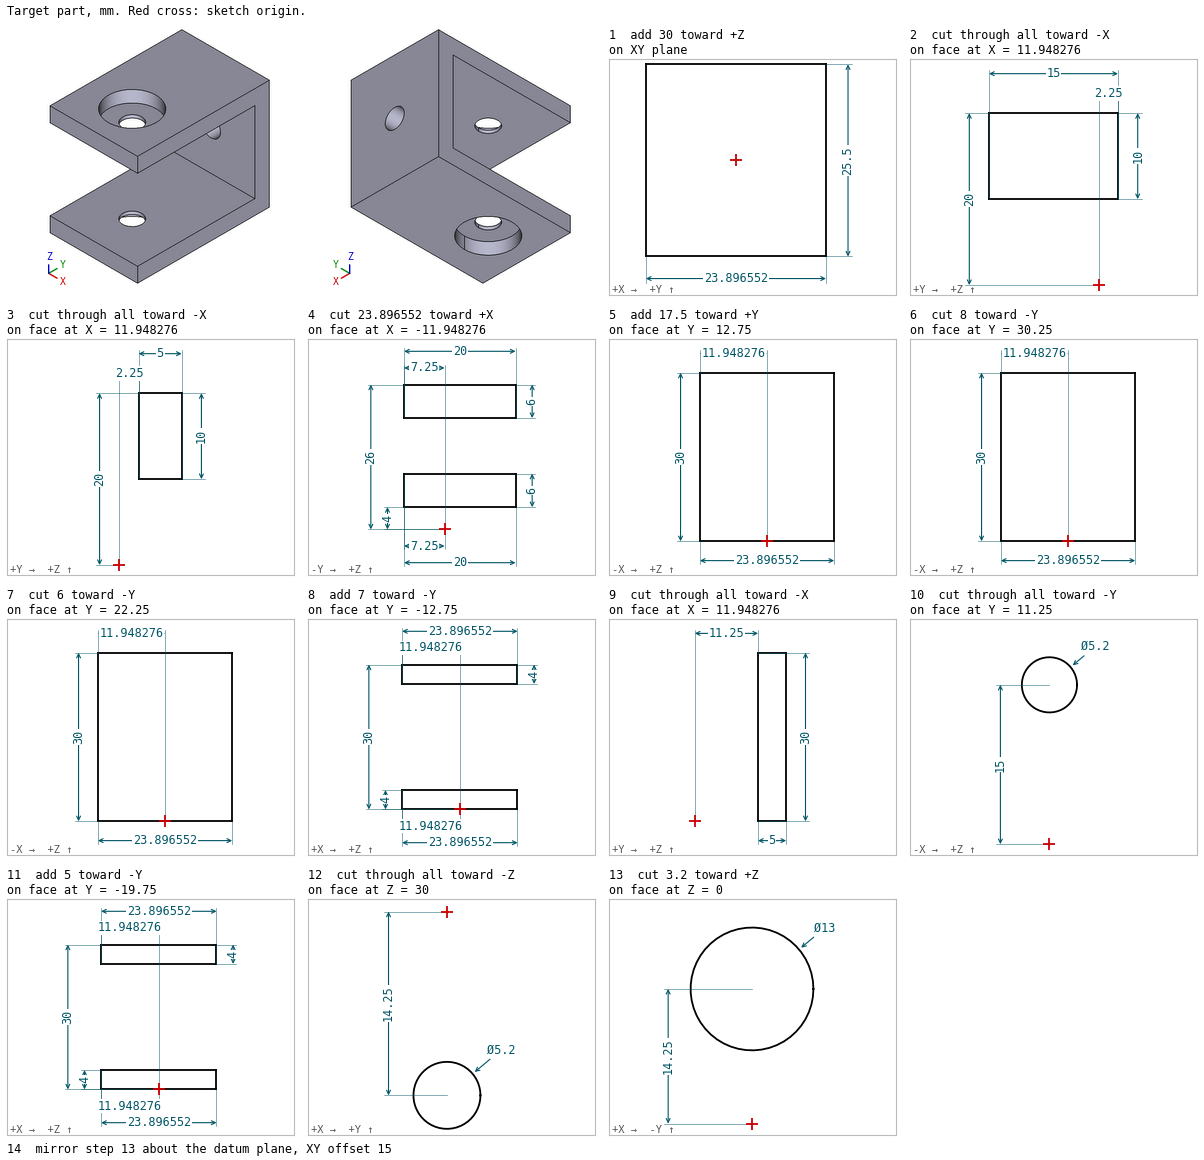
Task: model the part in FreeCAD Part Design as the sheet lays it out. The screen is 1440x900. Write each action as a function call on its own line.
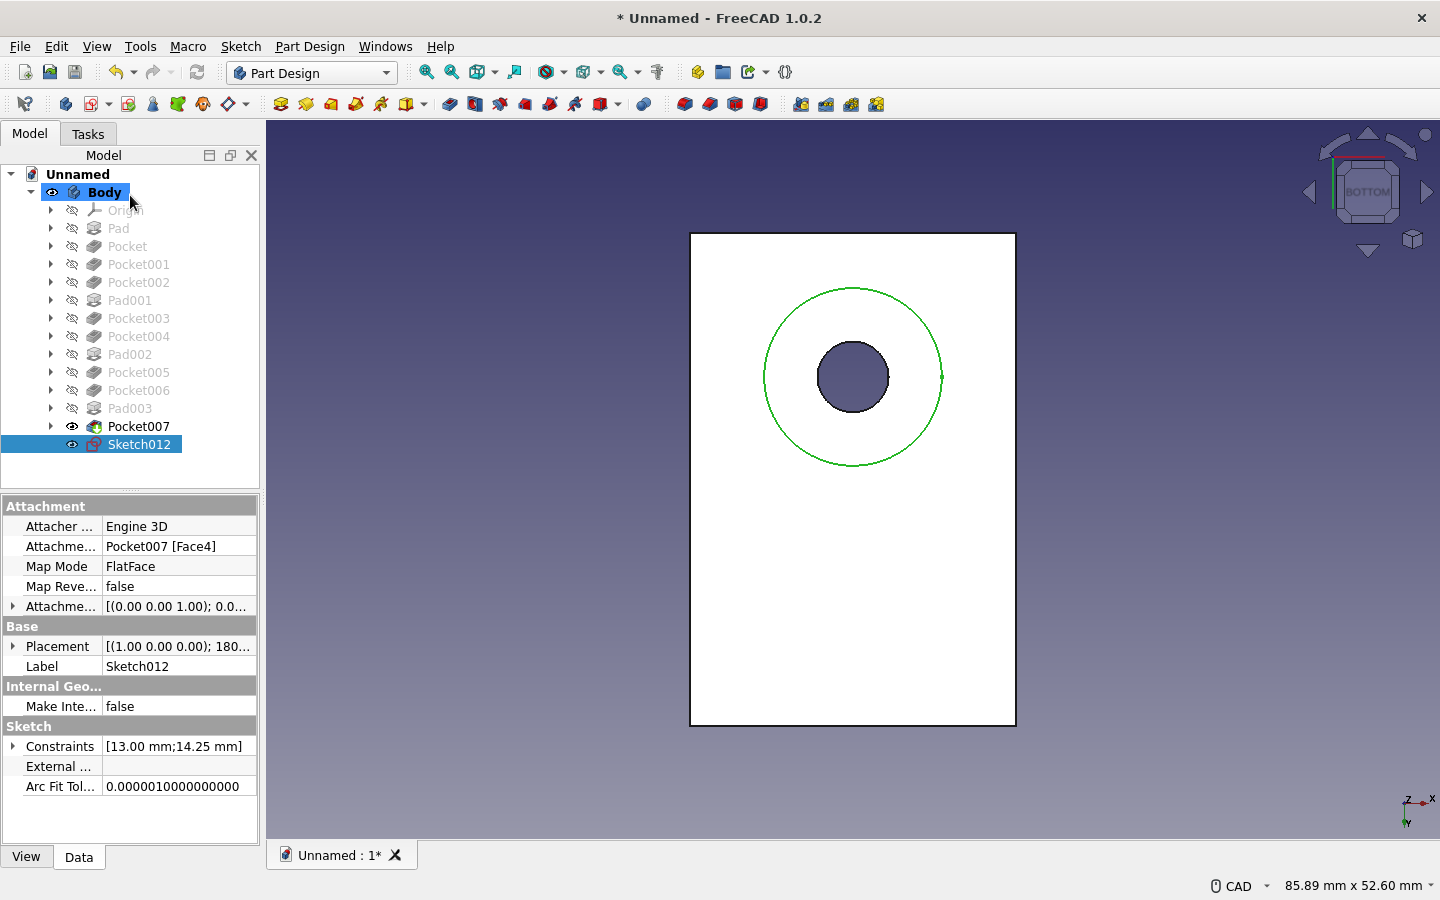
click(450, 104)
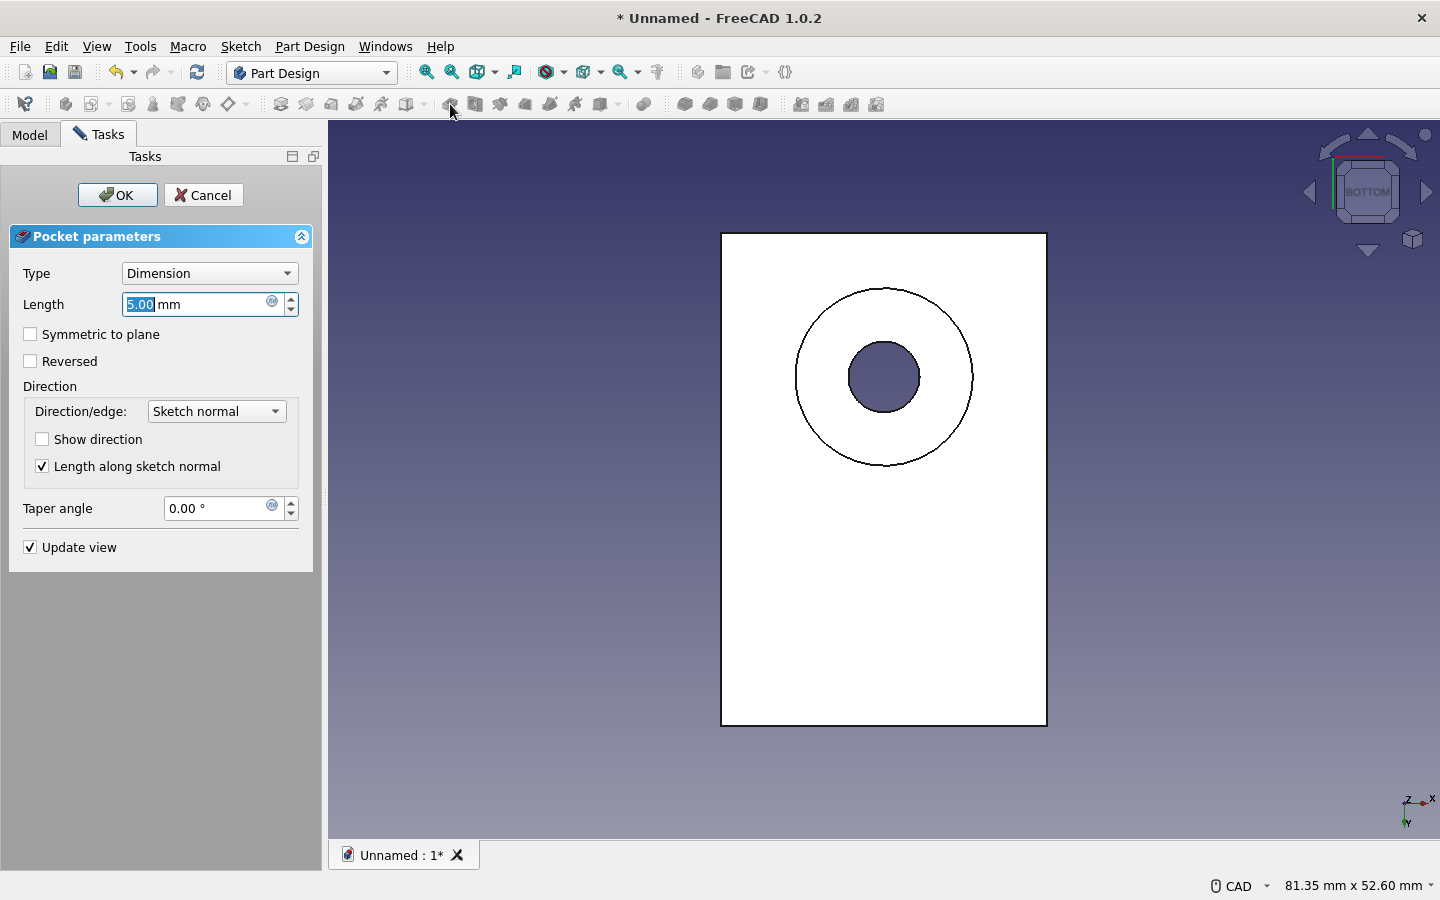
text(3.2)
key(Tab)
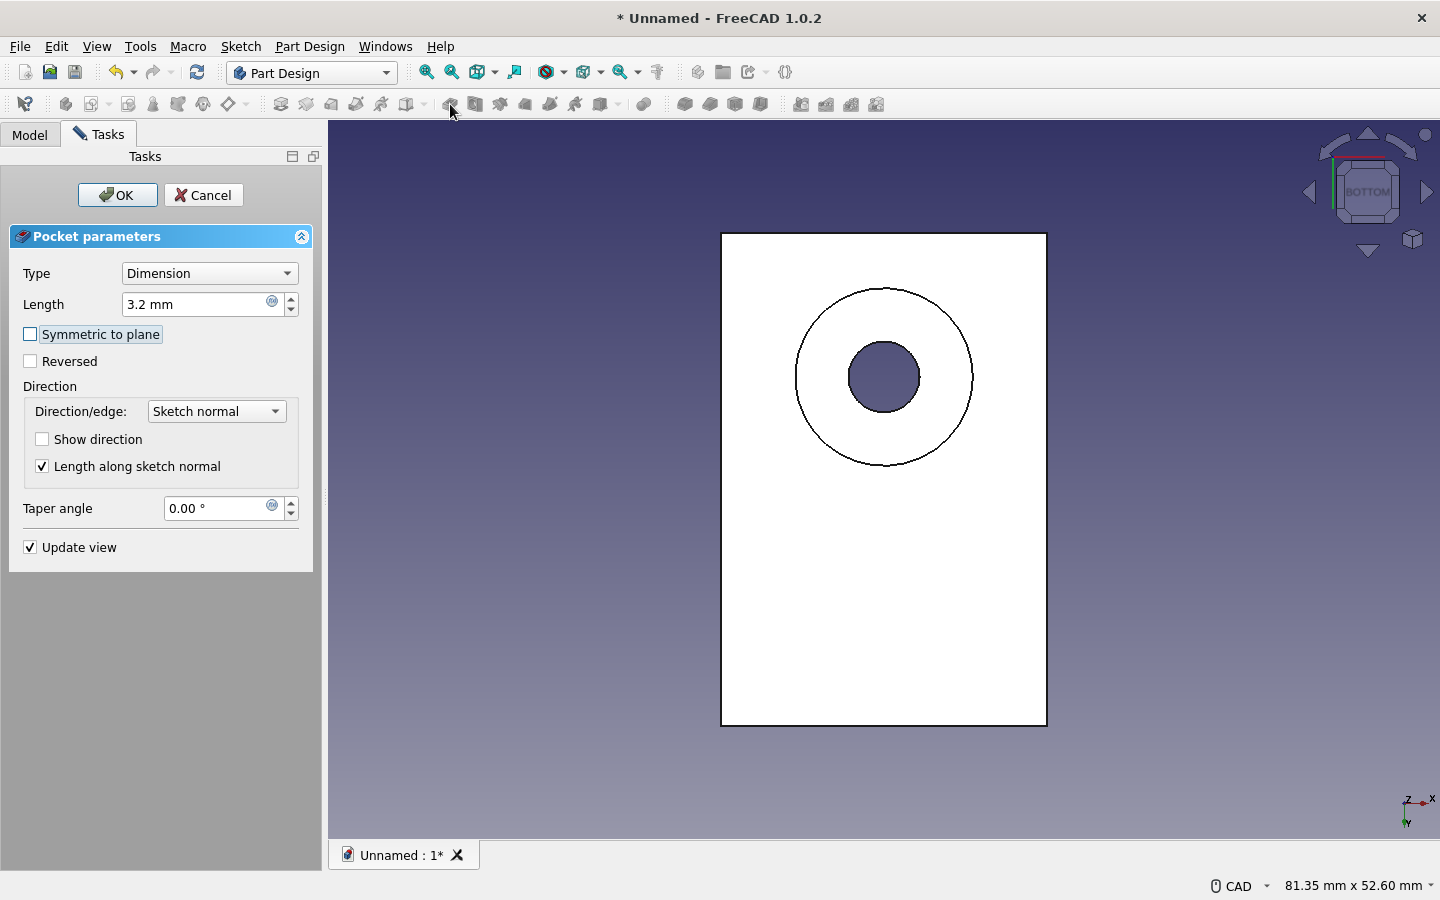
click(118, 195)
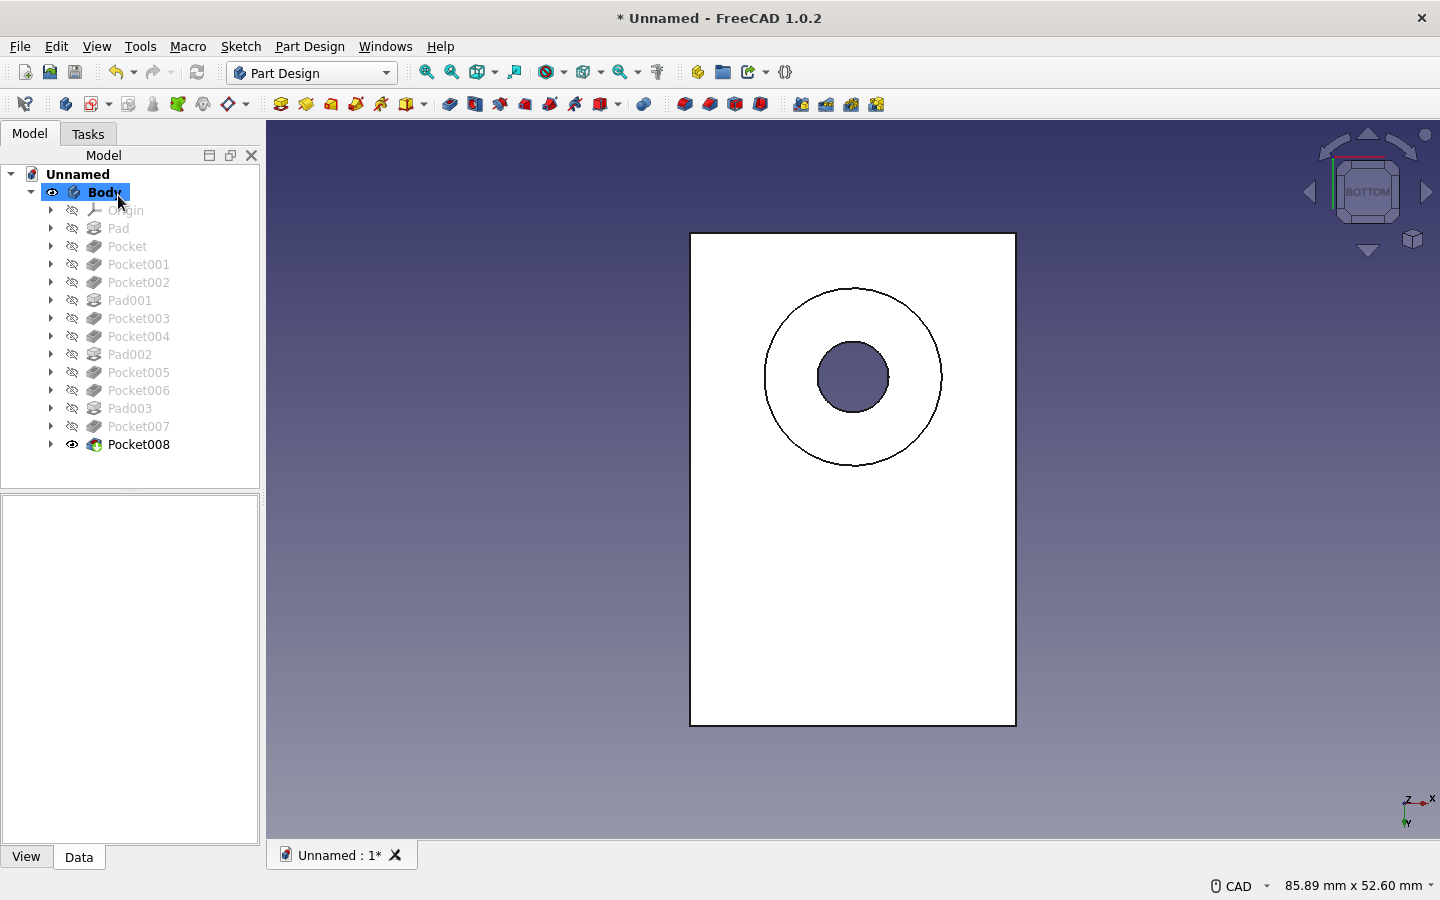
click(51, 210)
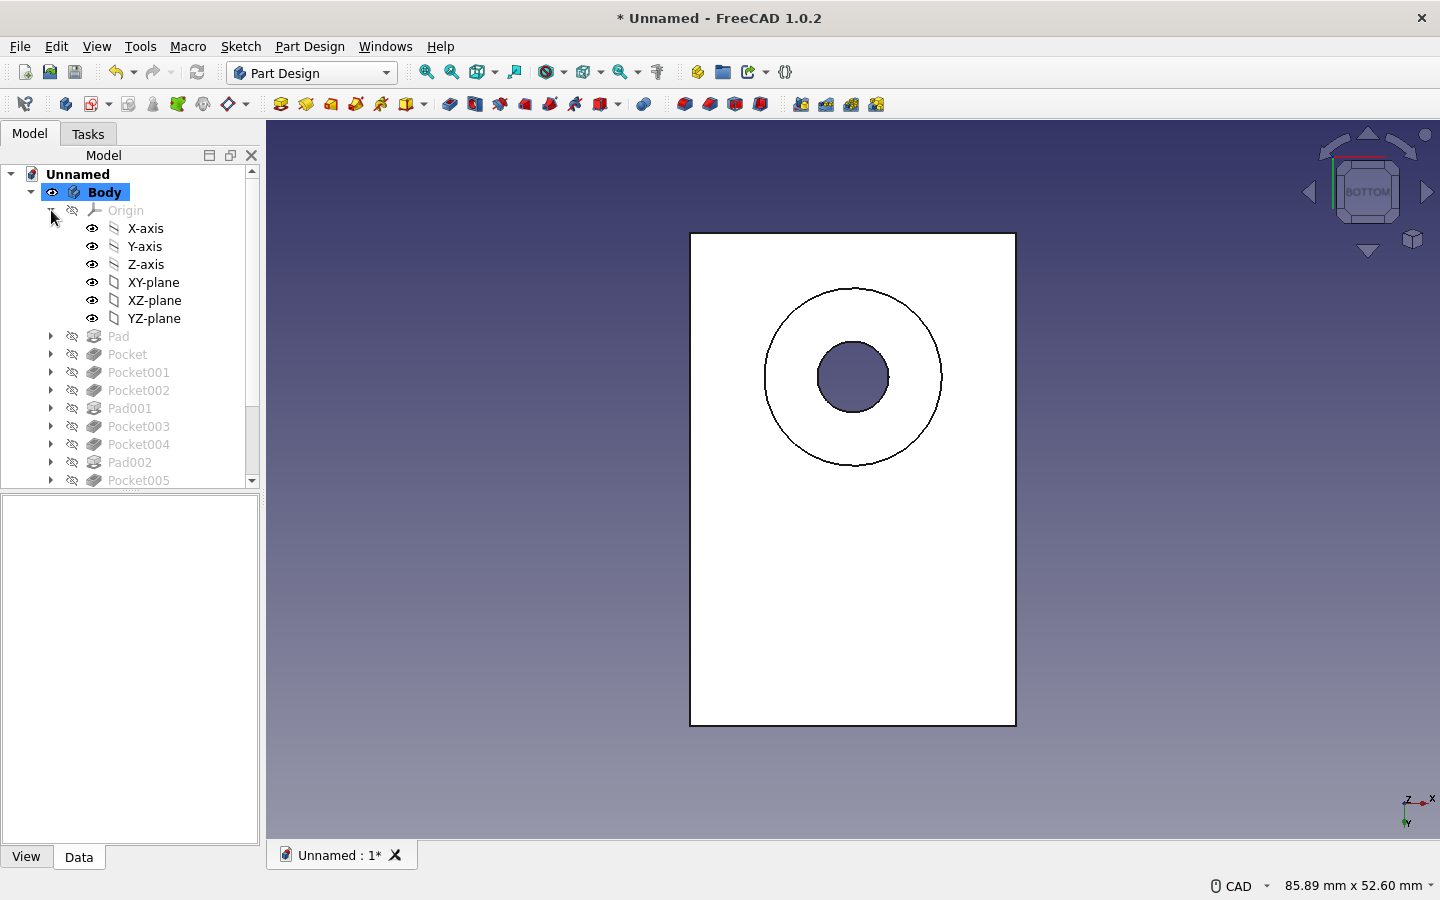
click(137, 282)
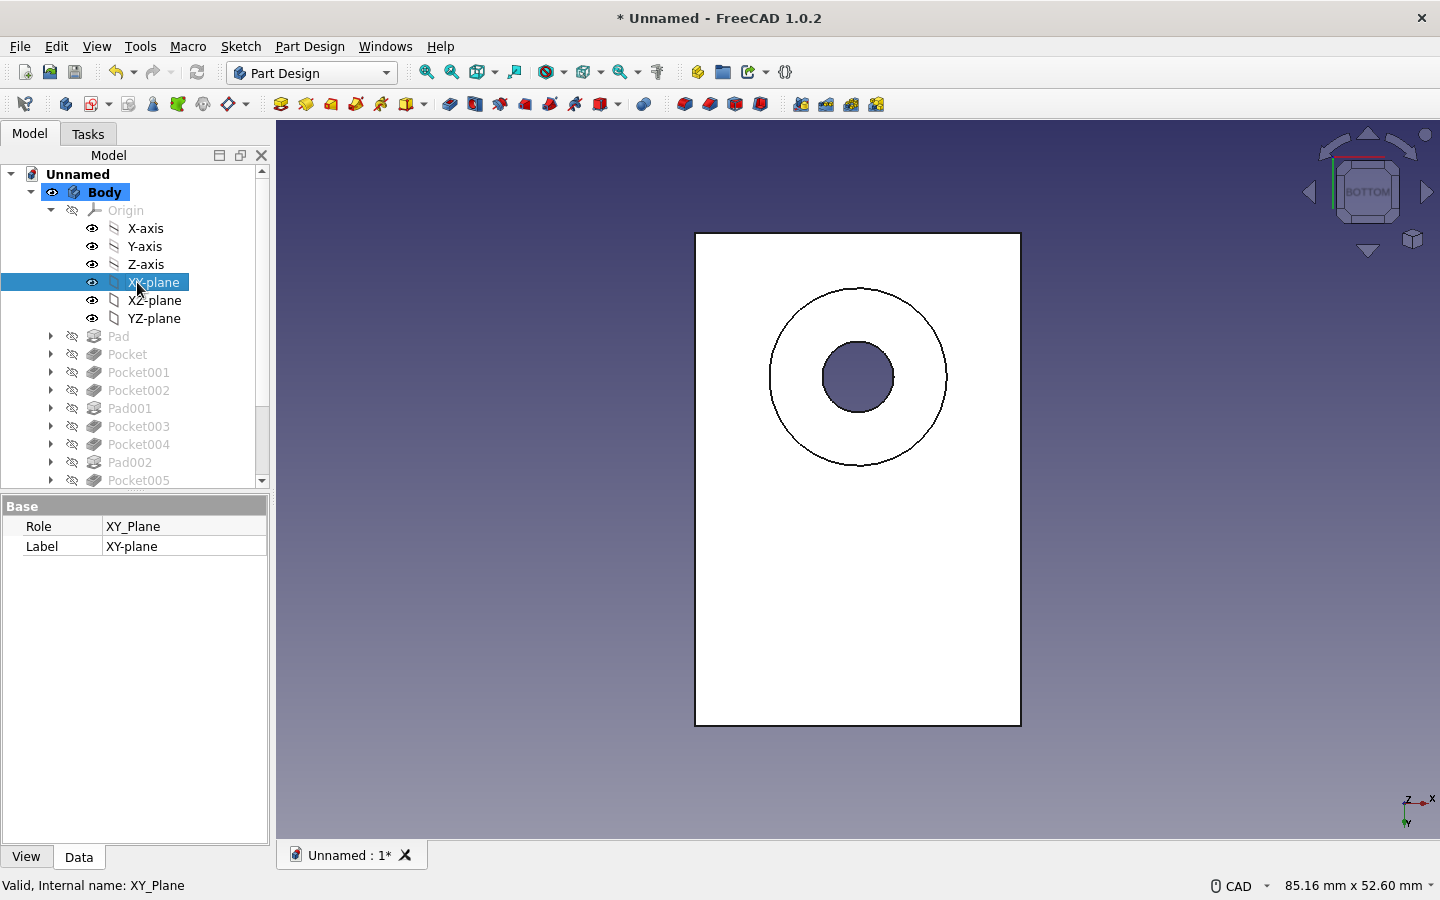
click(228, 104)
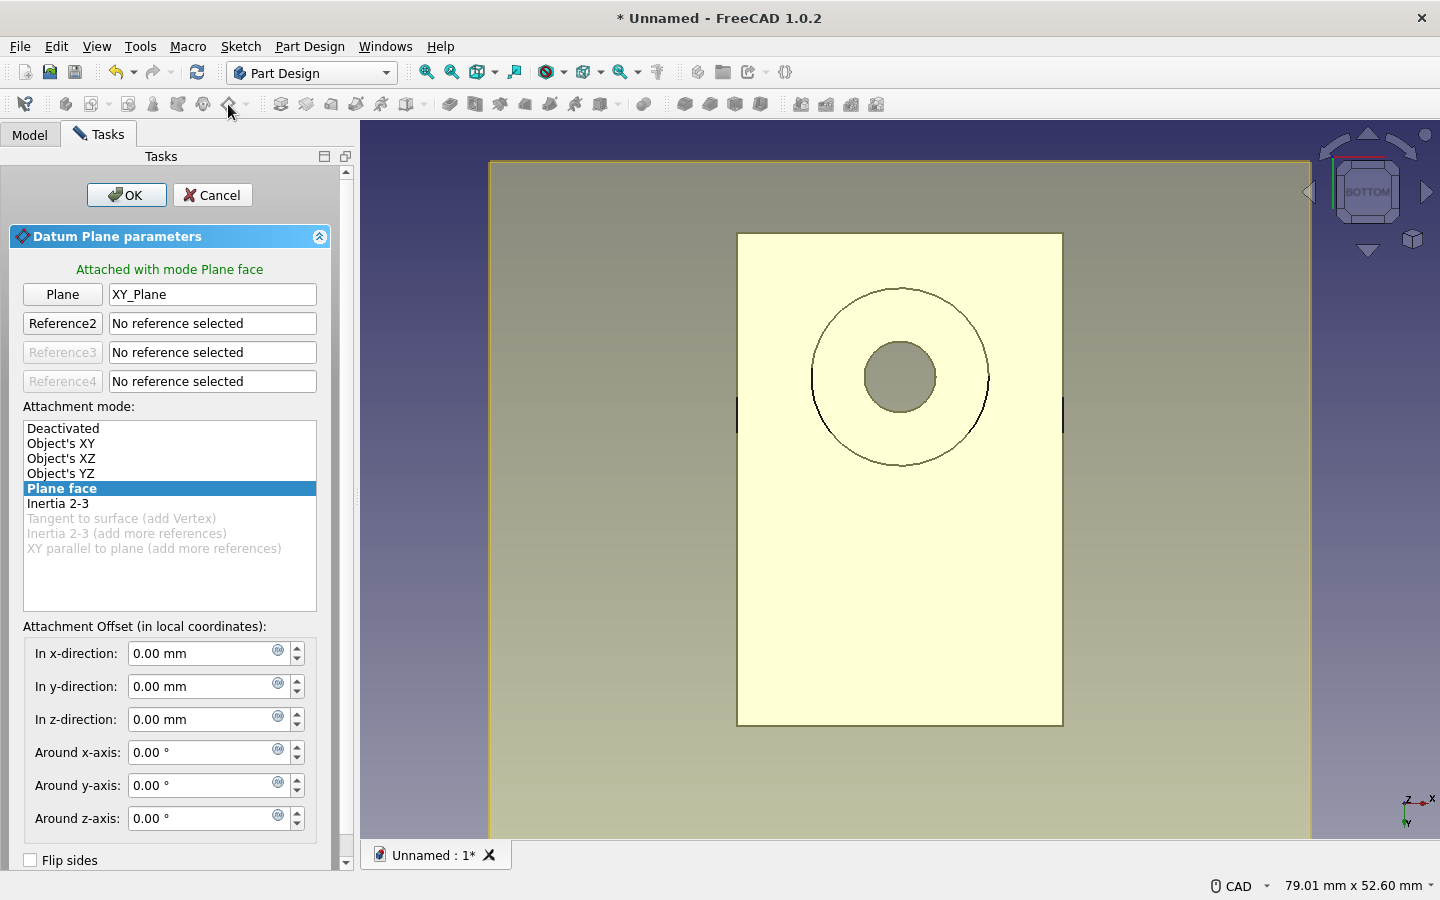
triple_click(210, 720)